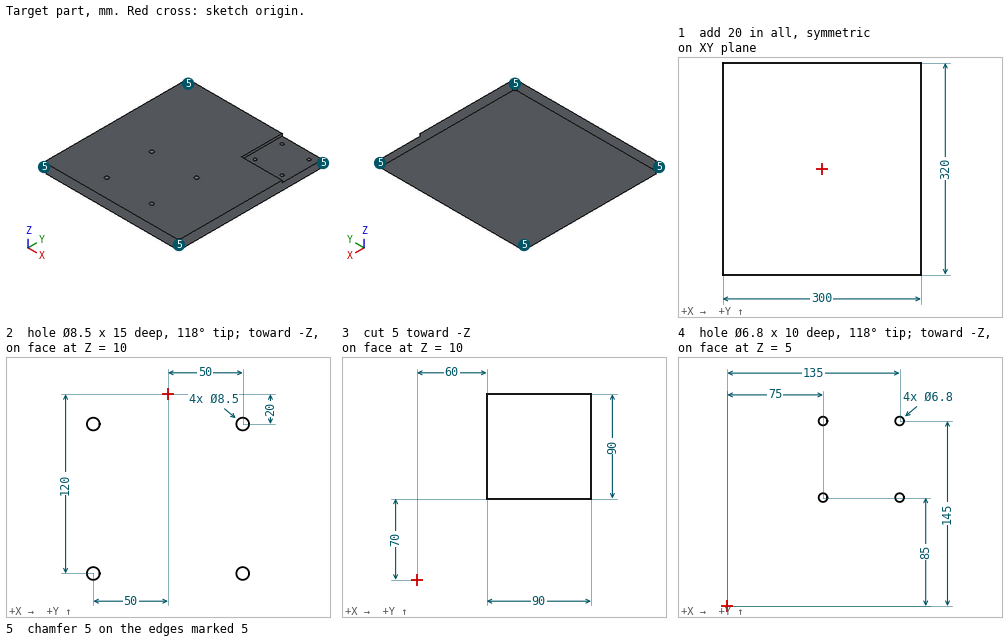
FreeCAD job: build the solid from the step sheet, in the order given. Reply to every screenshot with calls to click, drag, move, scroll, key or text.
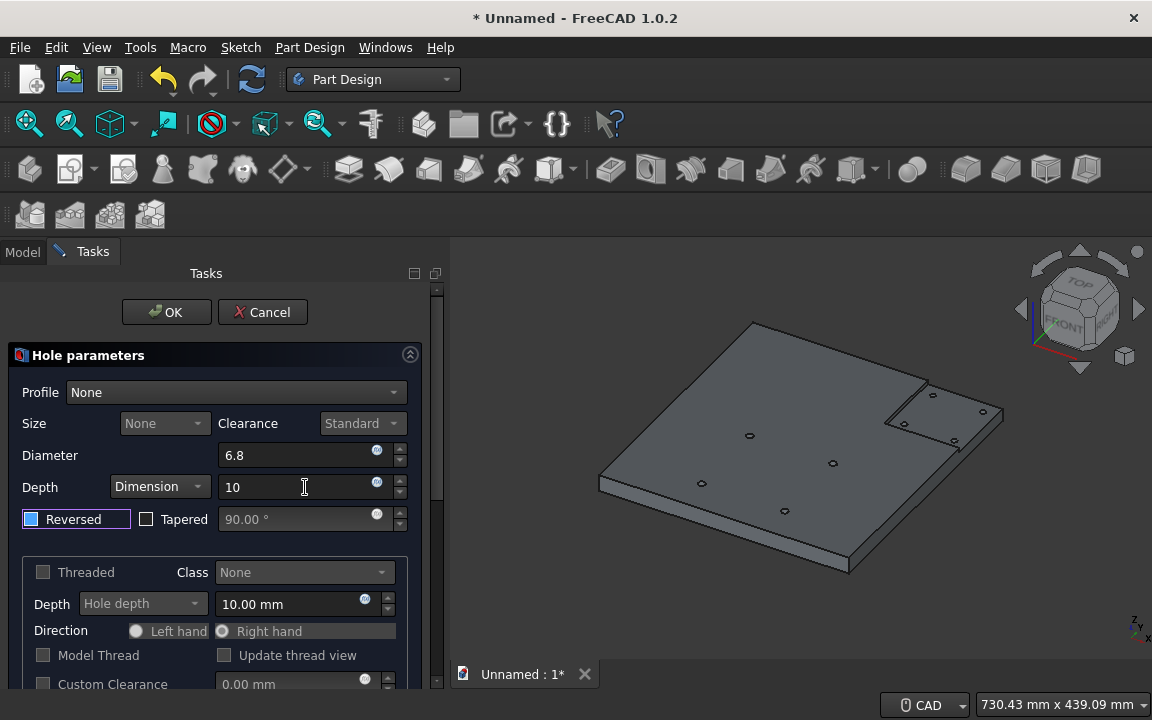
click(167, 312)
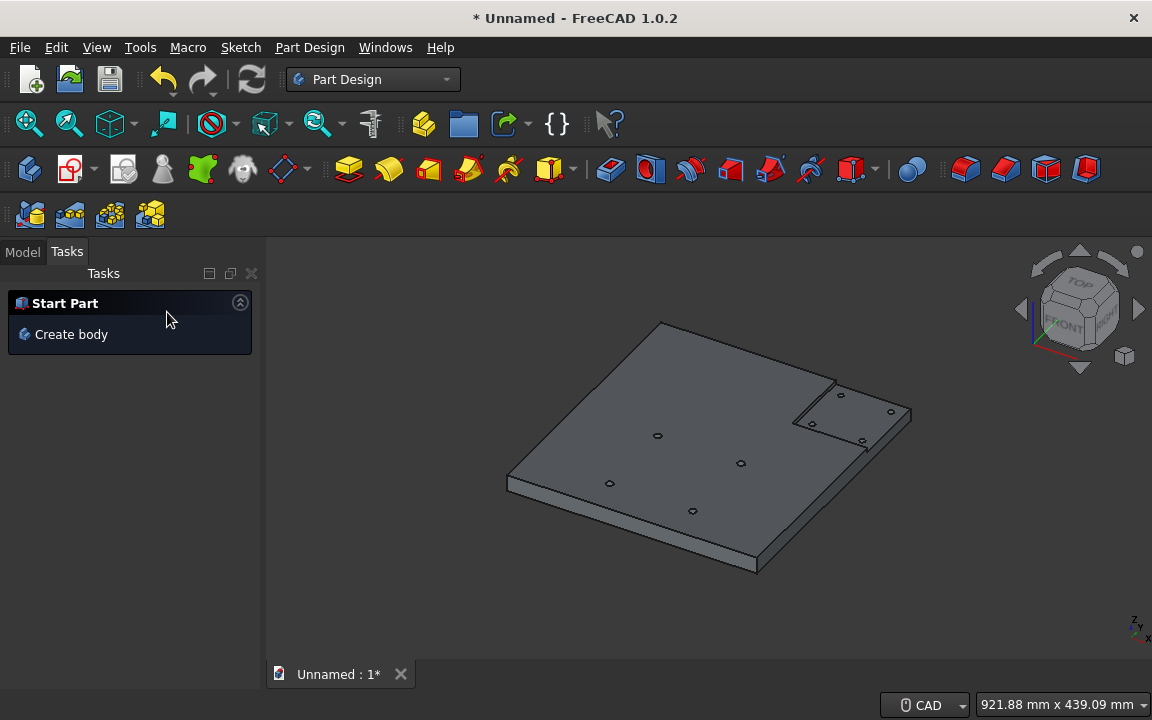
click(757, 565)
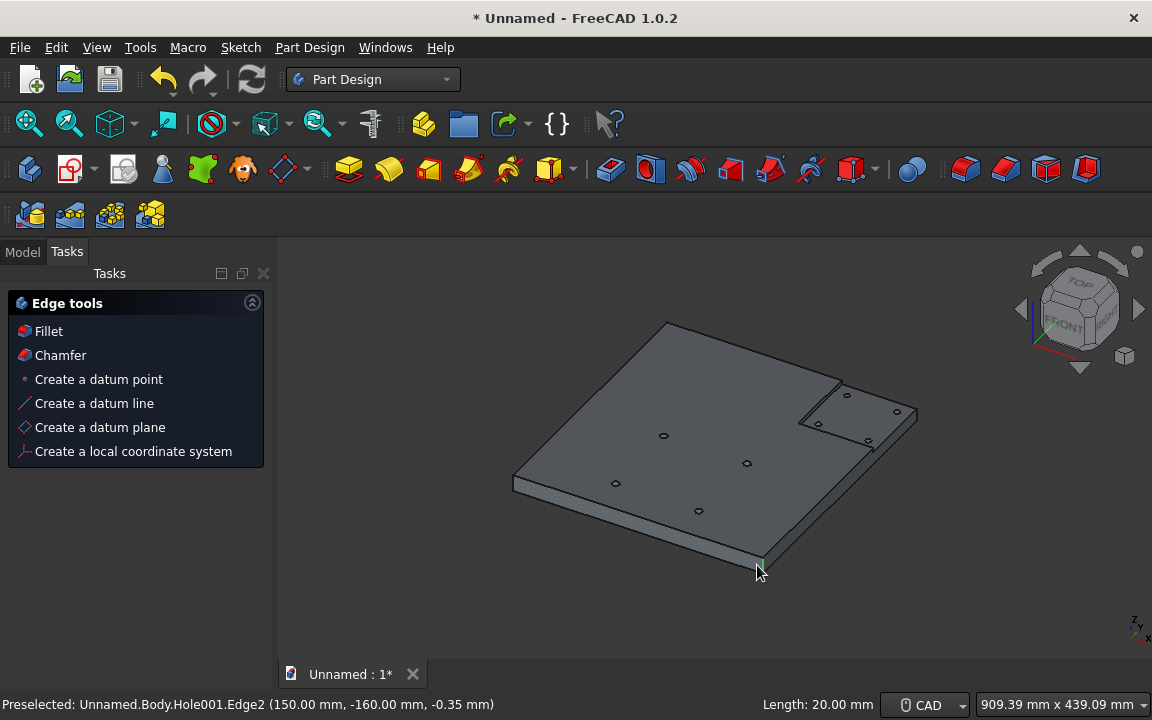
scroll(917, 414, up, 6)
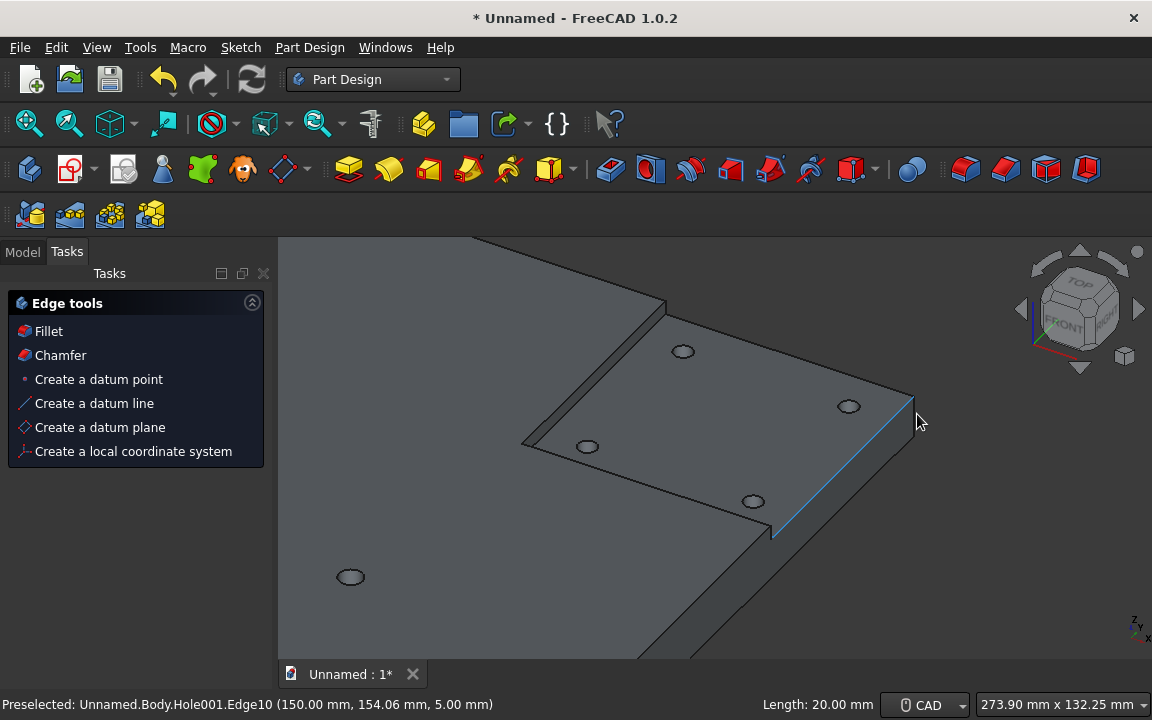
click(30, 124)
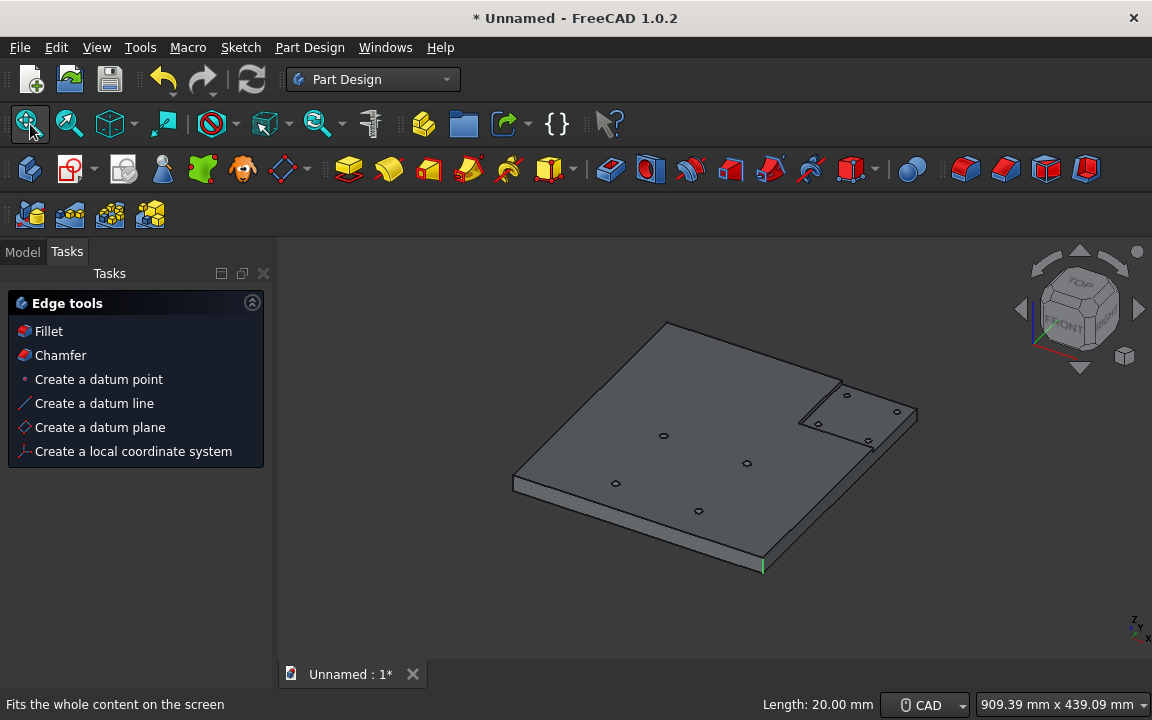
key(0)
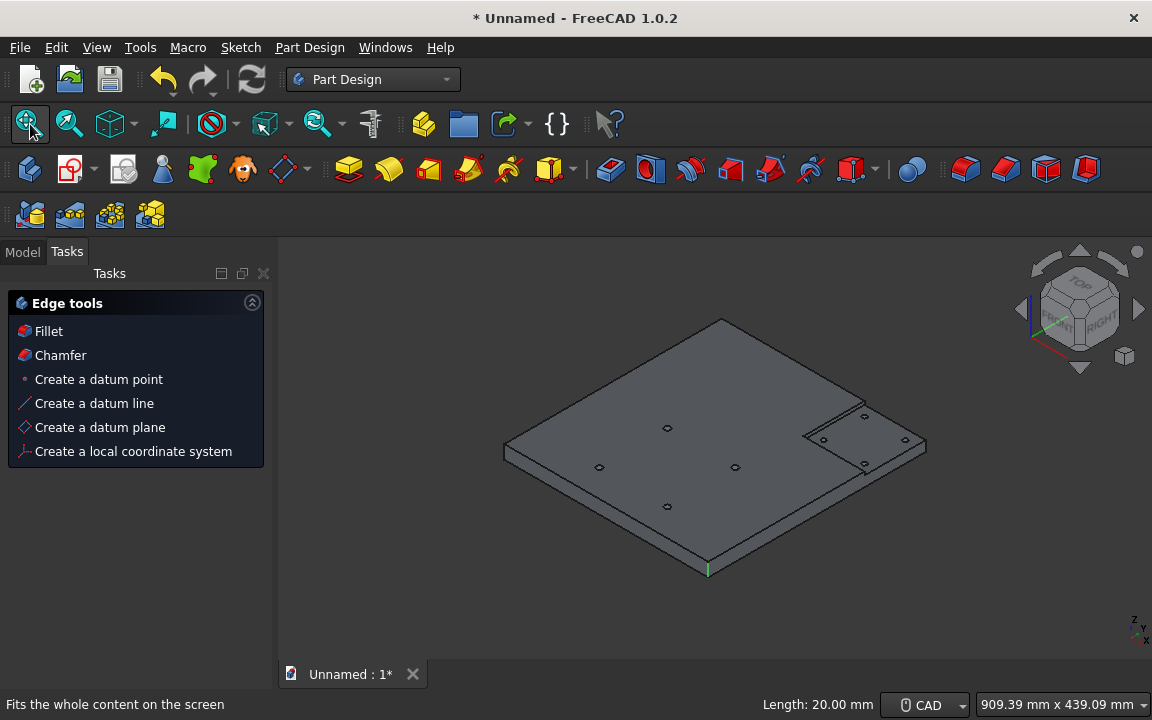
scroll(926, 445, up, 6)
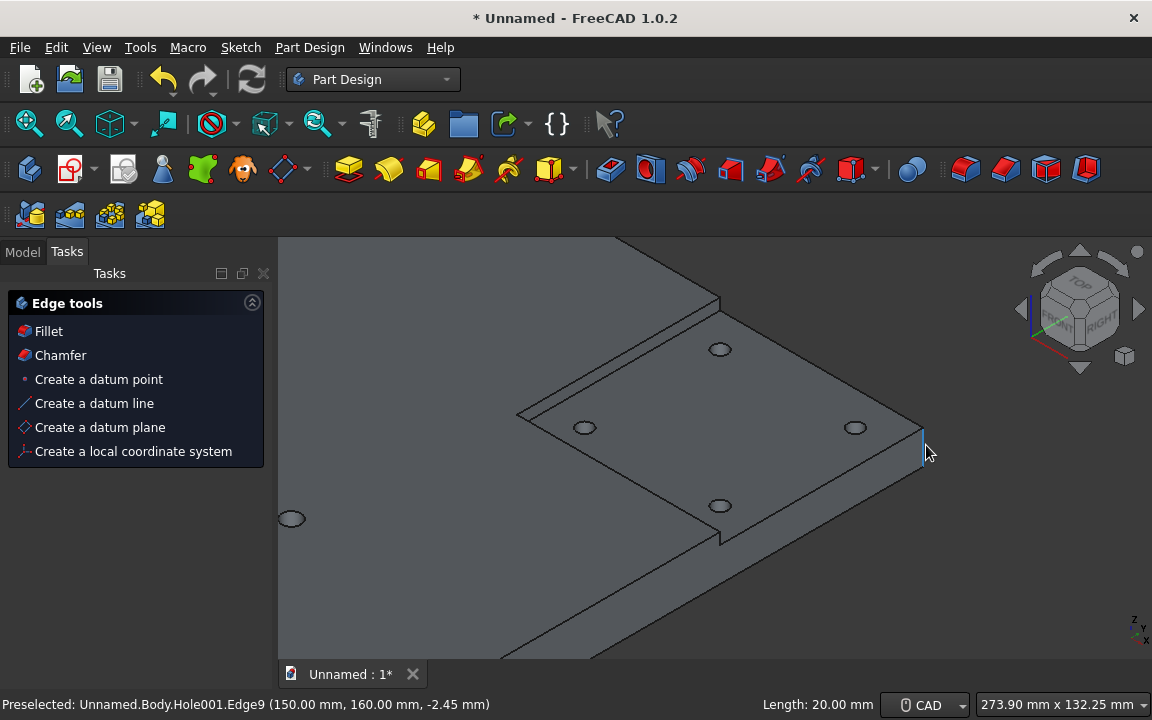
click(30, 124)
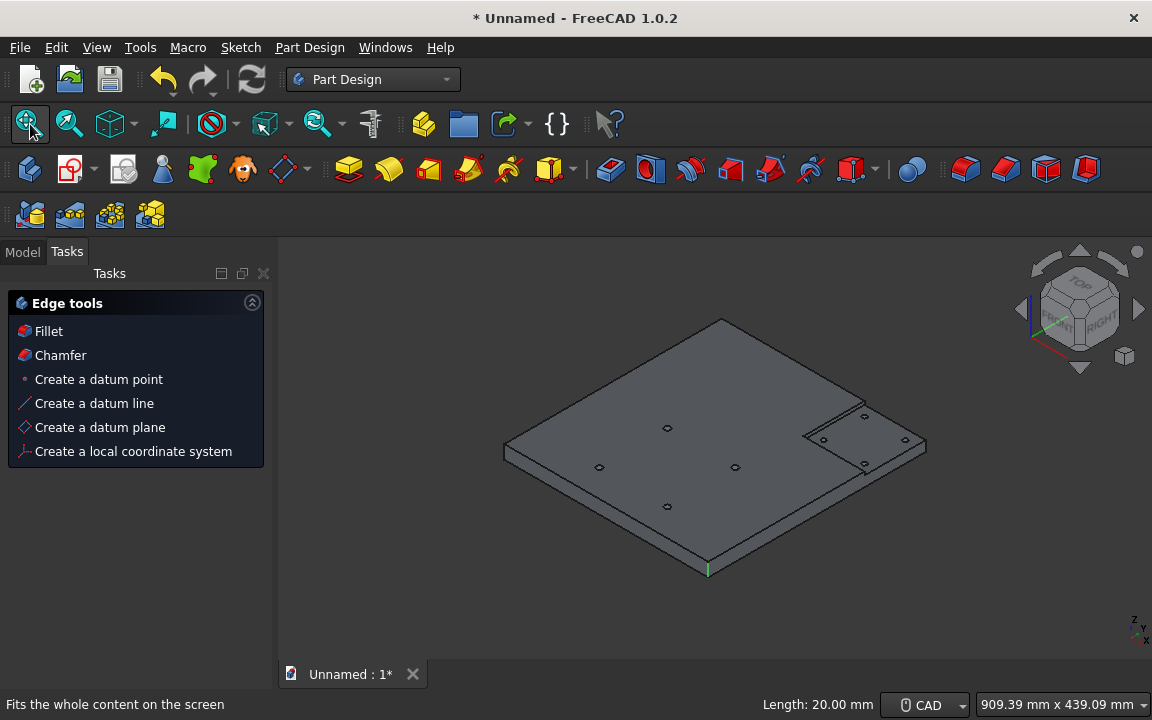
key(2)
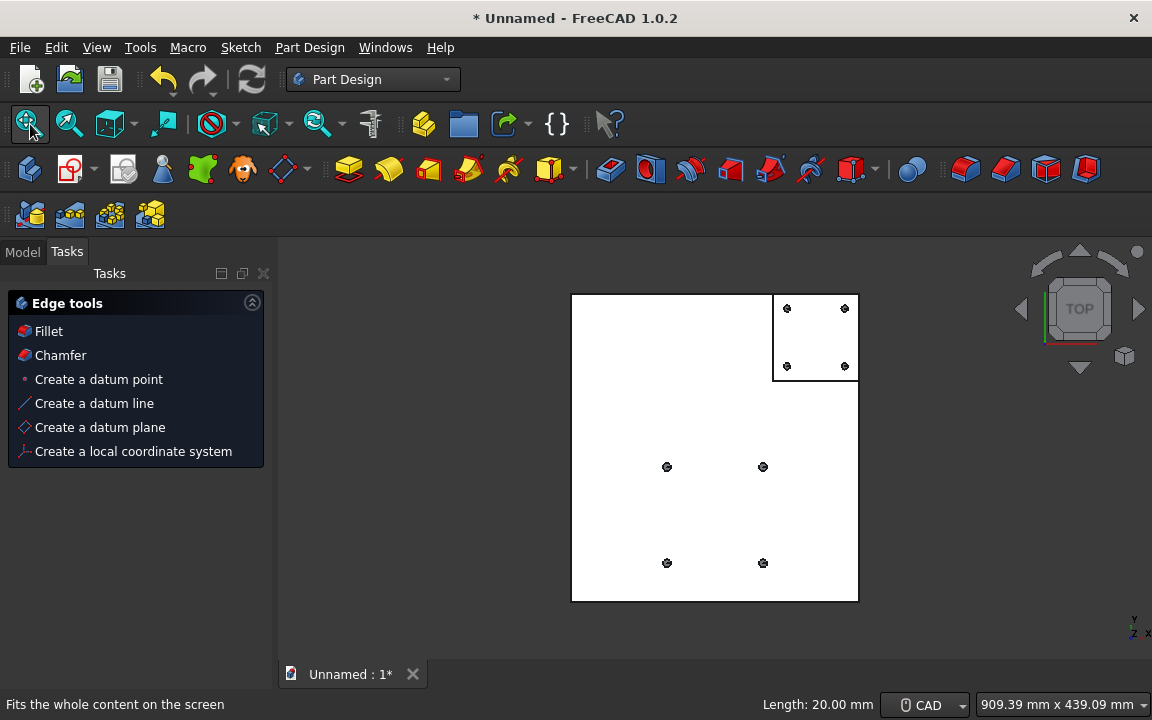
scroll(859, 293, up, 6)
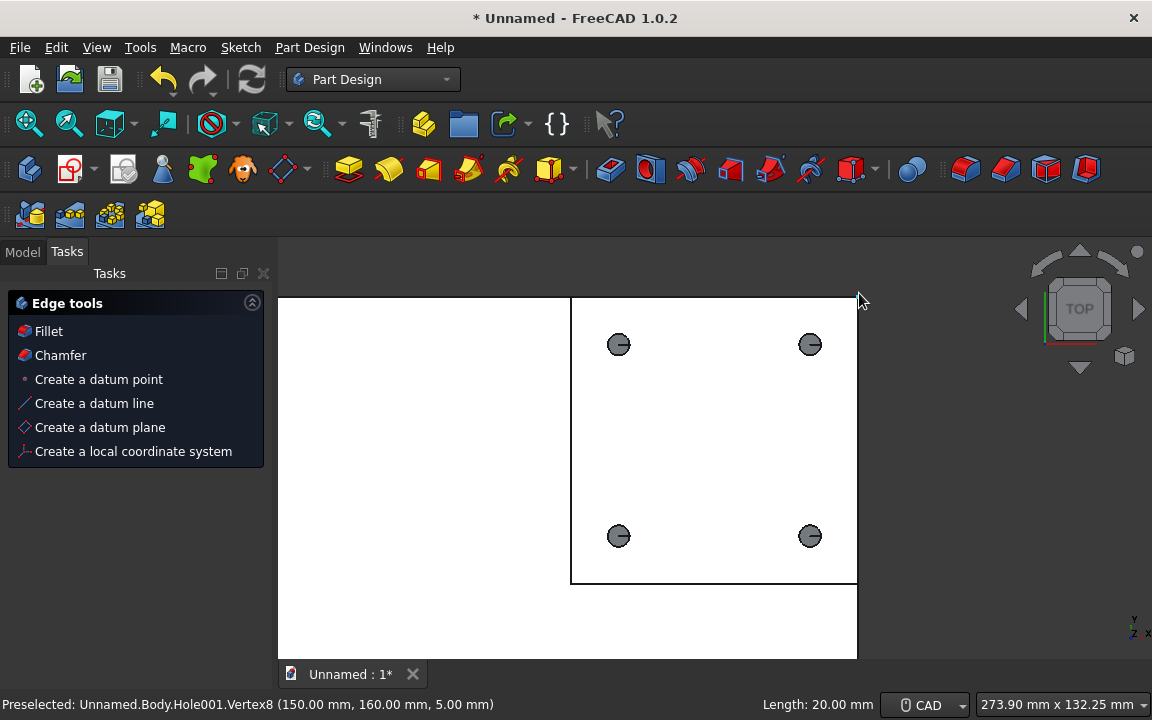
key(v)
key(f)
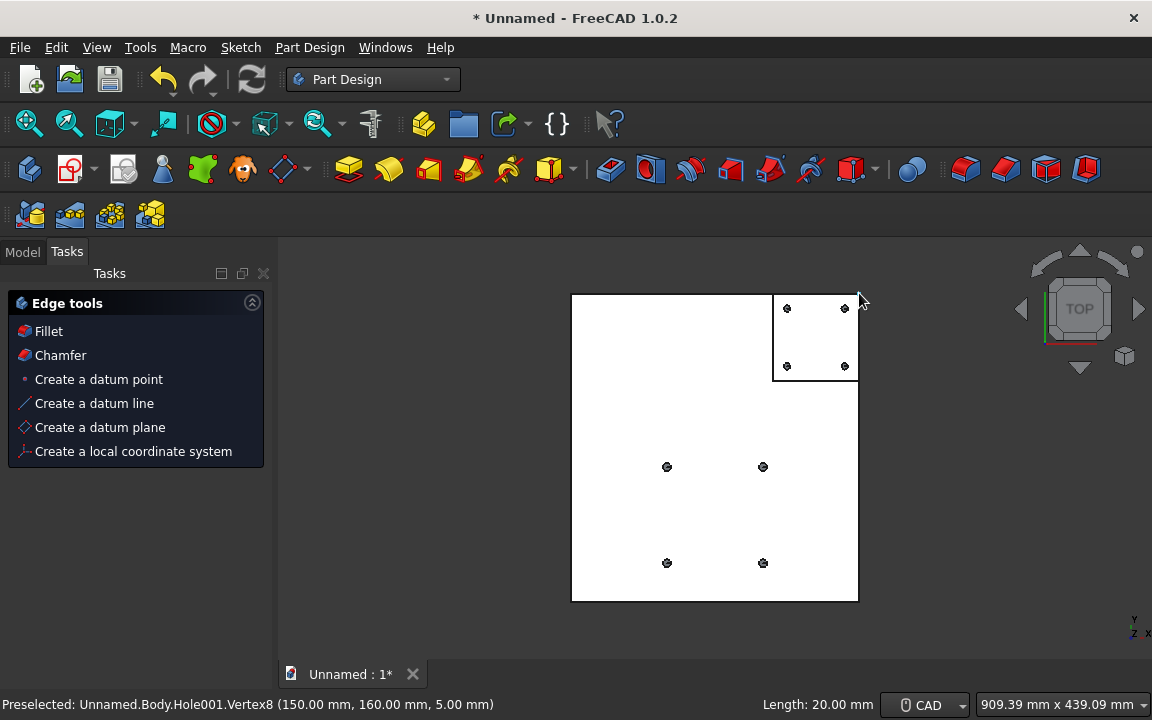
key(1)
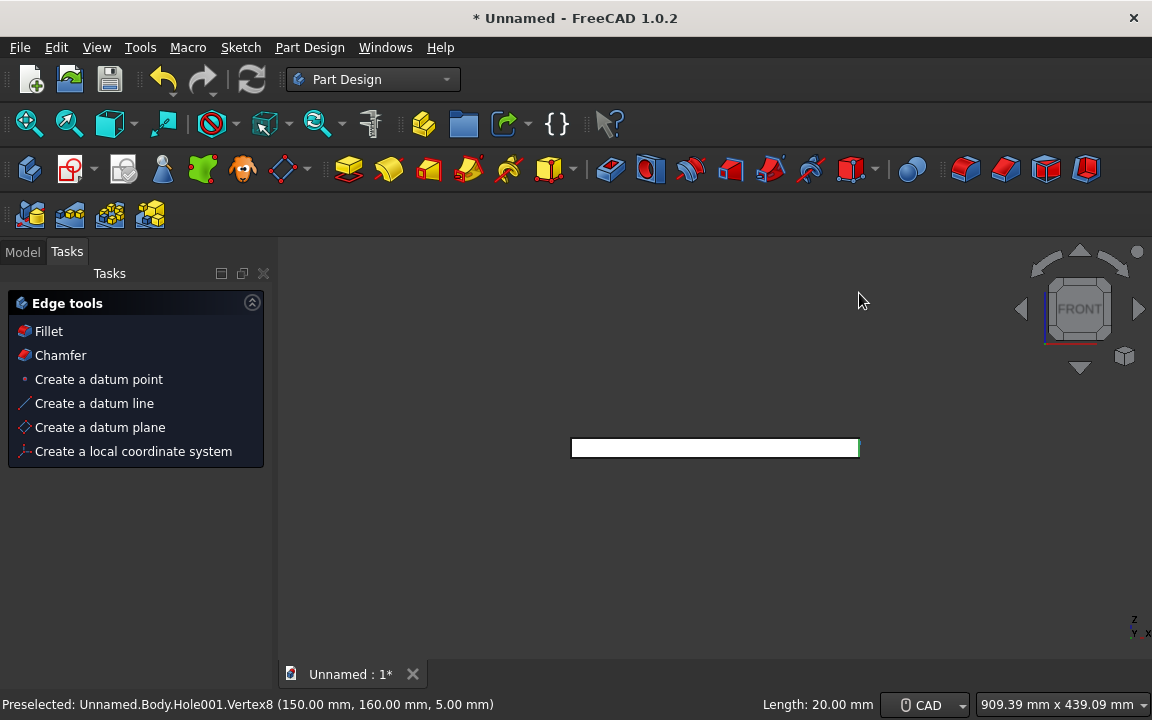
key(v)
key(f)